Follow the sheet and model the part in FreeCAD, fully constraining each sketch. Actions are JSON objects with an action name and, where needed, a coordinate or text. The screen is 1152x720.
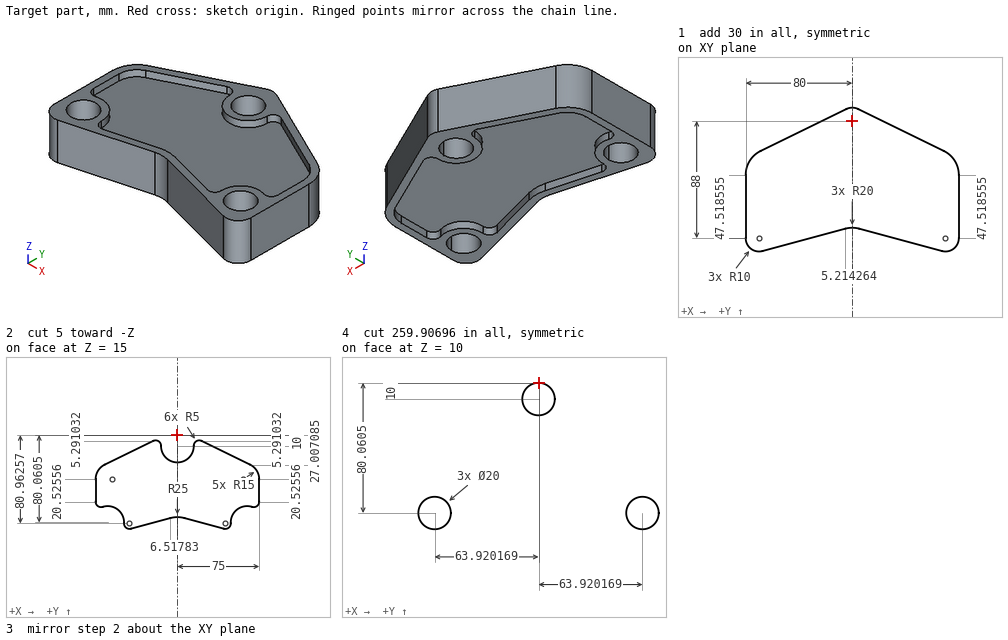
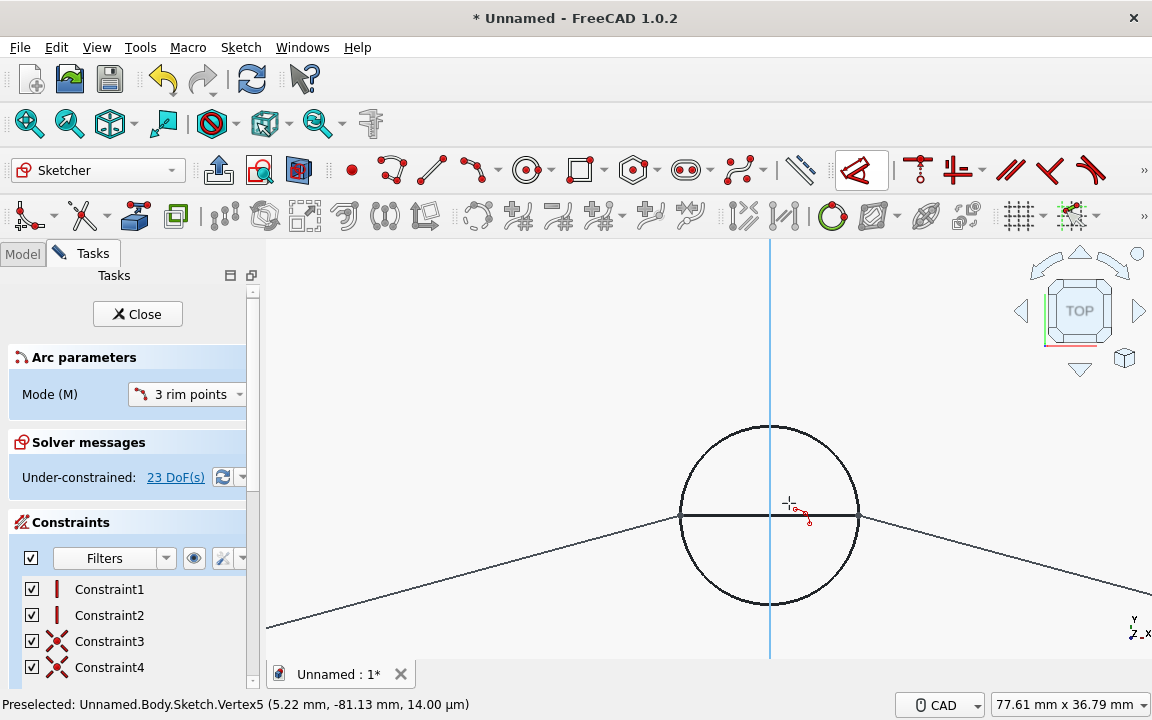
{"action": "left_click", "coordinate": [787, 498]}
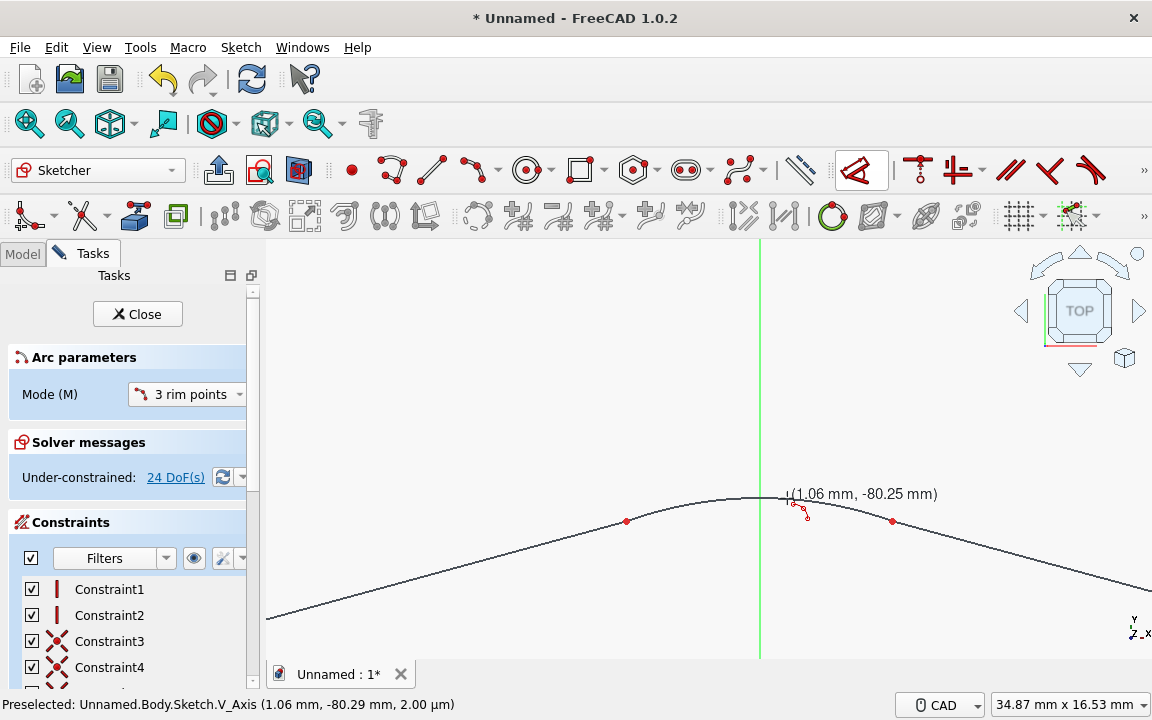
{"action": "scroll", "coordinate": [629, 536], "scroll_direction": "down", "scroll_amount": 12}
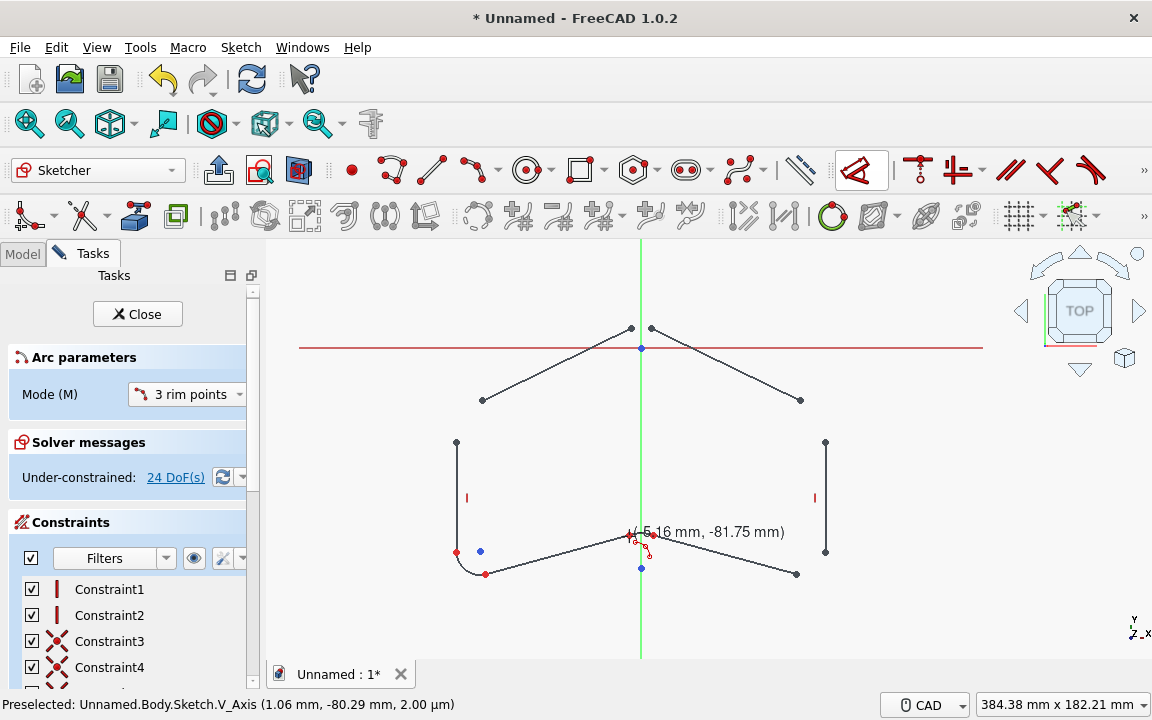
{"action": "left_click", "coordinate": [797, 574]}
{"action": "left_click", "coordinate": [826, 552]}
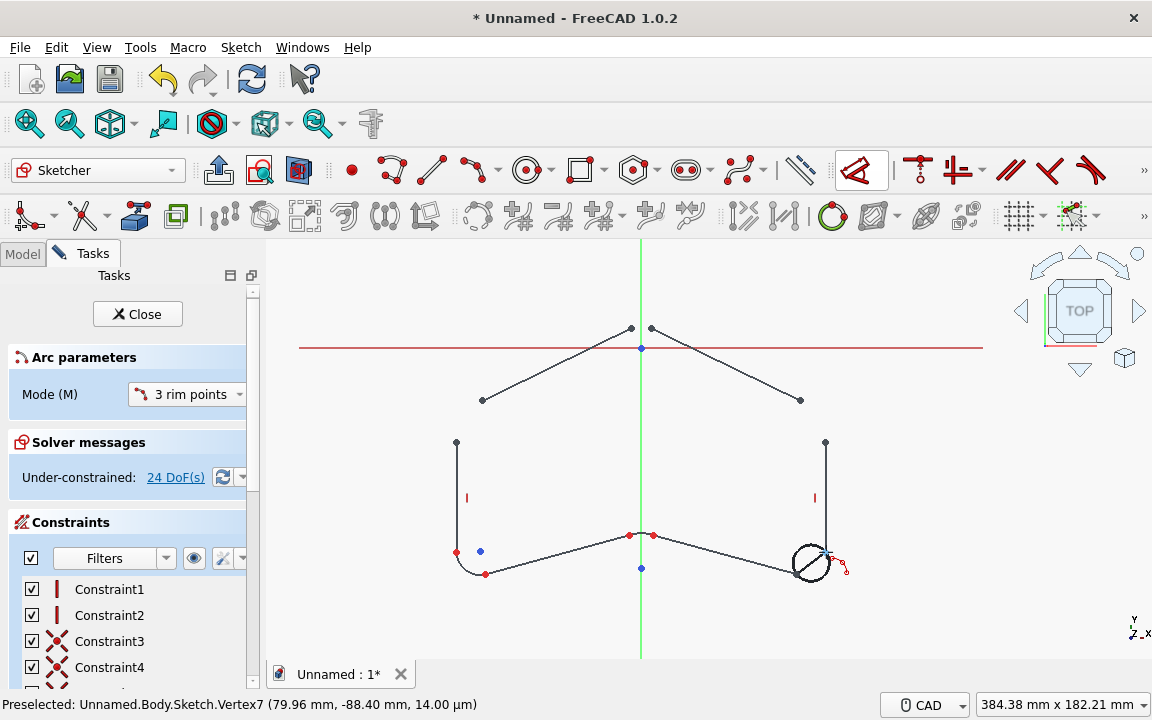
{"action": "scroll", "coordinate": [817, 569], "scroll_direction": "up", "scroll_amount": 3}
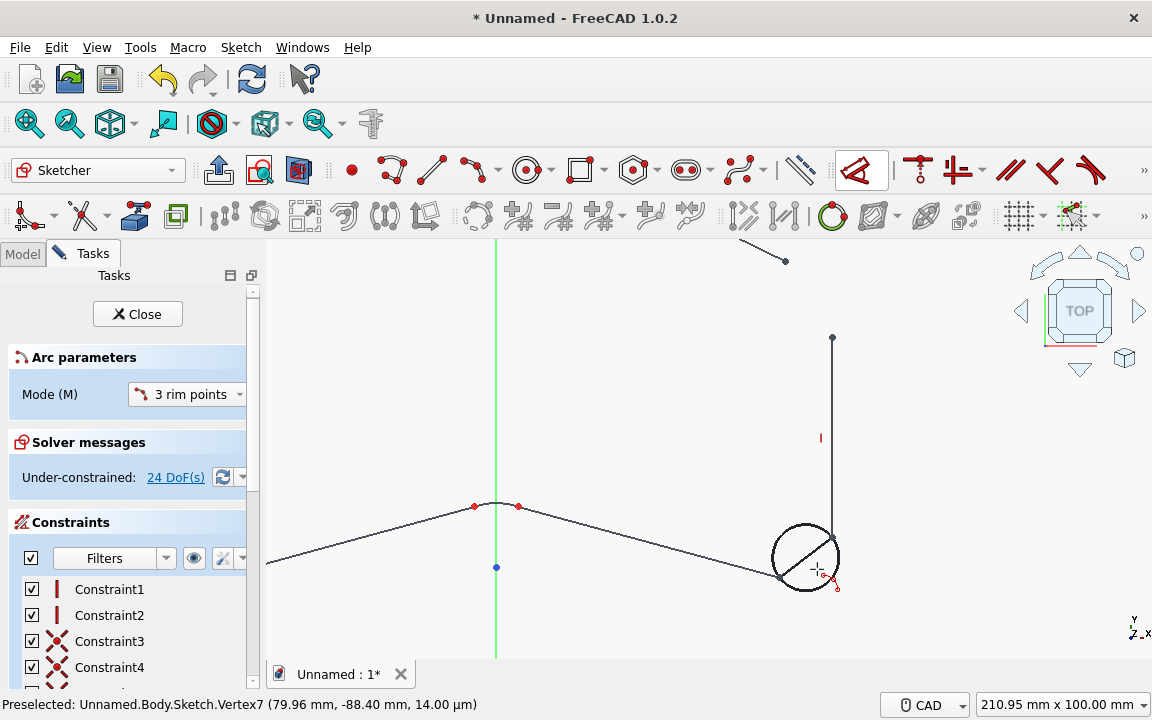
{"action": "left_click", "coordinate": [816, 569]}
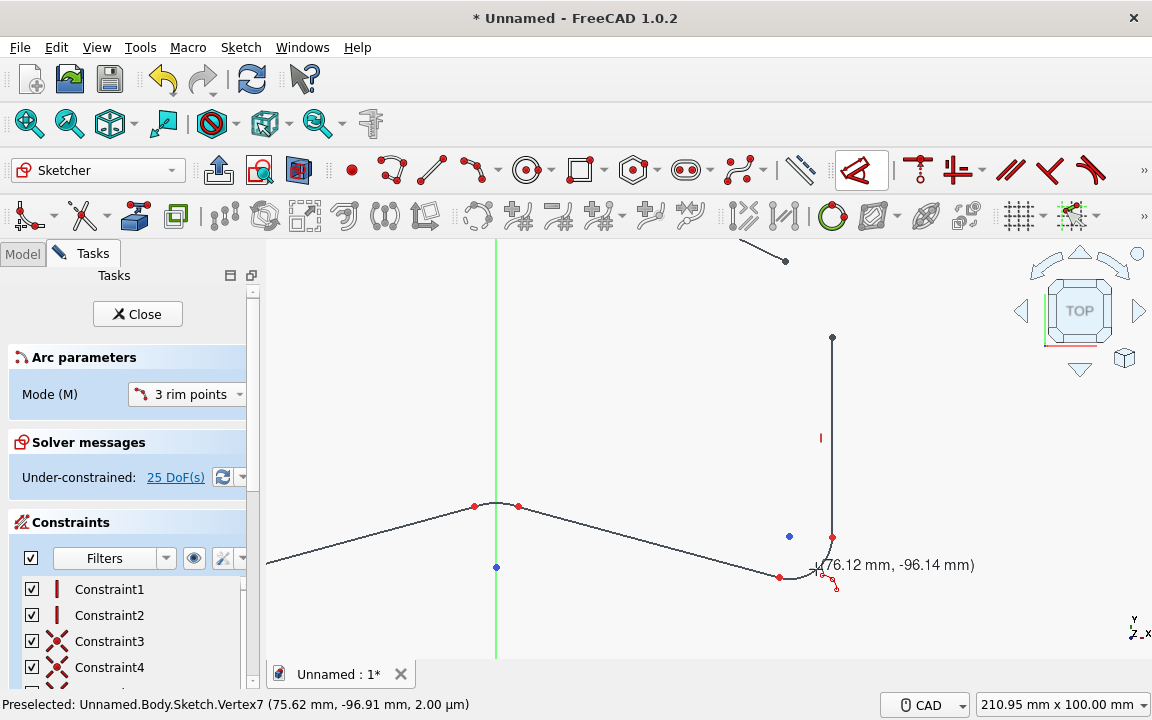
{"action": "left_click", "coordinate": [832, 337]}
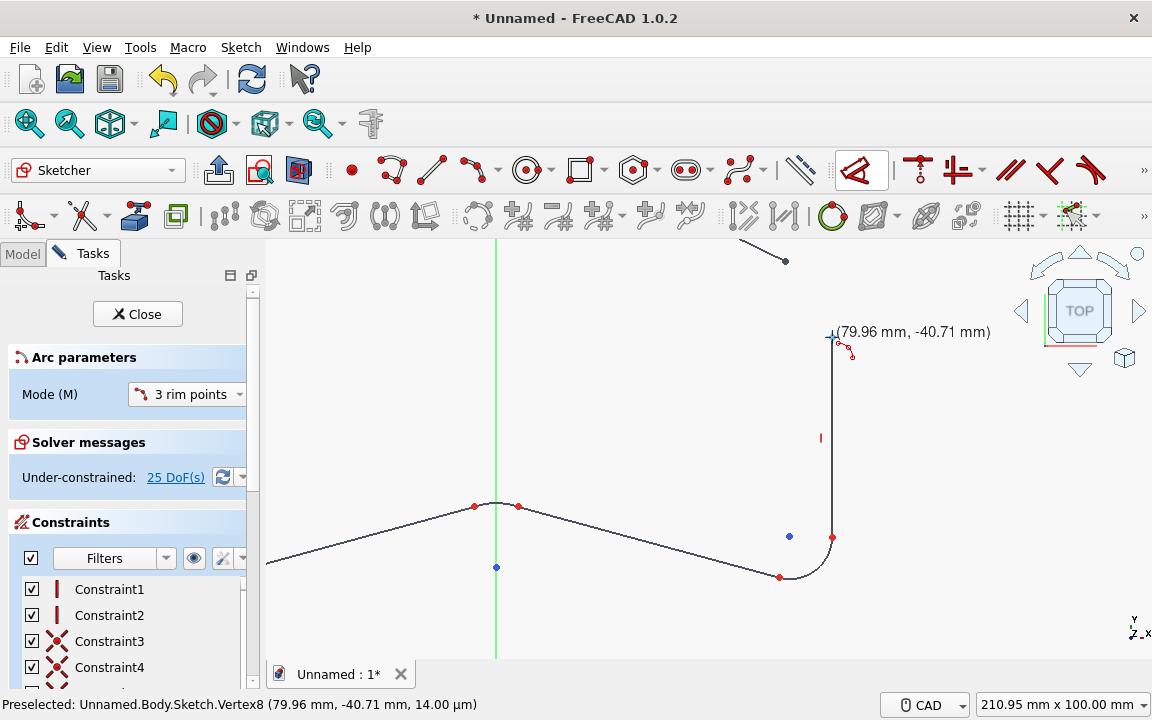
{"action": "scroll", "coordinate": [816, 569], "scroll_direction": "down", "scroll_amount": 3}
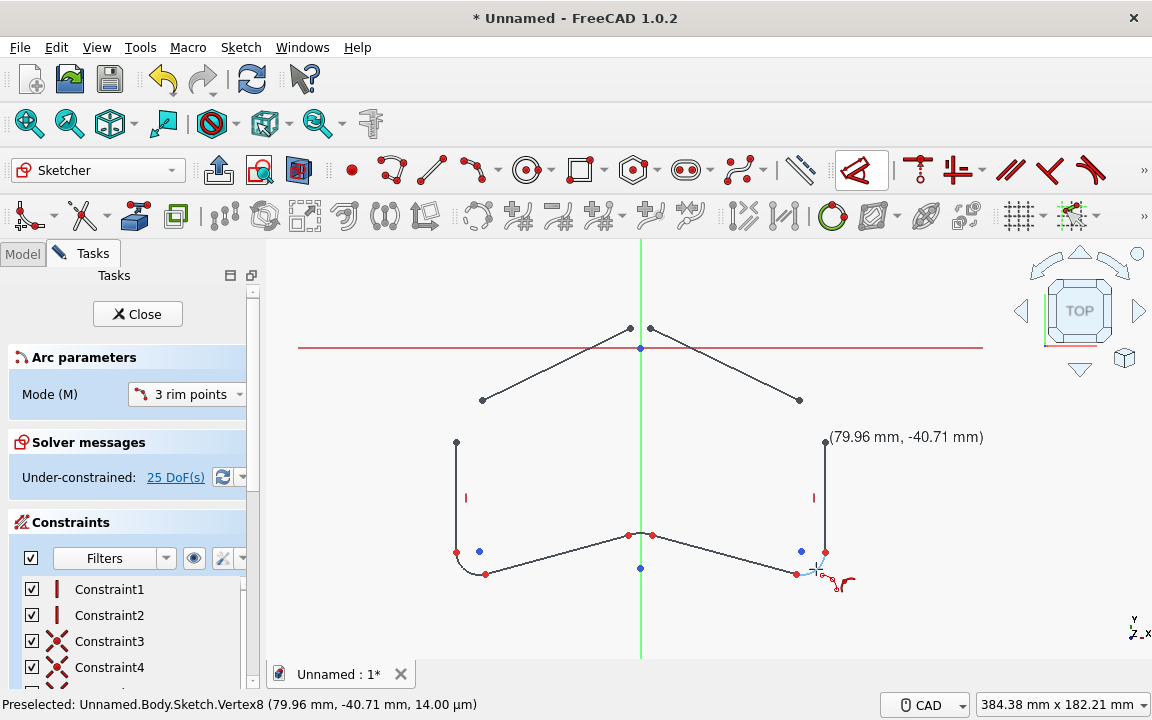
{"action": "left_click", "coordinate": [800, 401]}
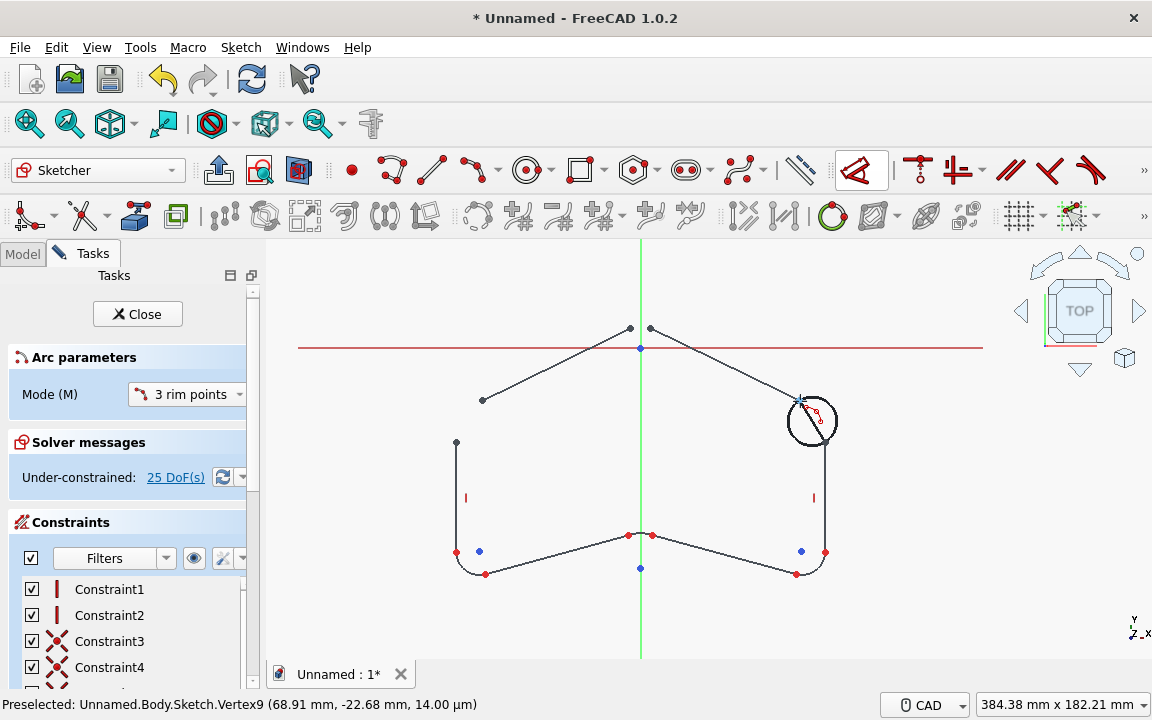
{"action": "scroll", "coordinate": [818, 417], "scroll_direction": "up", "scroll_amount": 5}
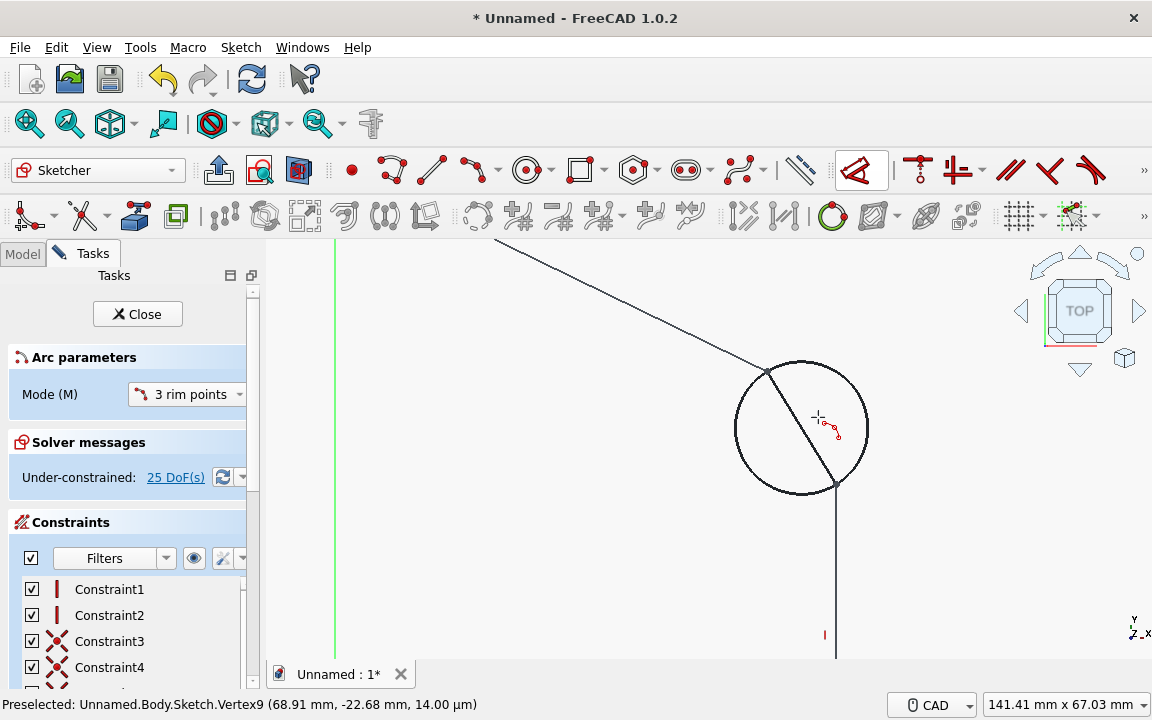
{"action": "left_click", "coordinate": [818, 417]}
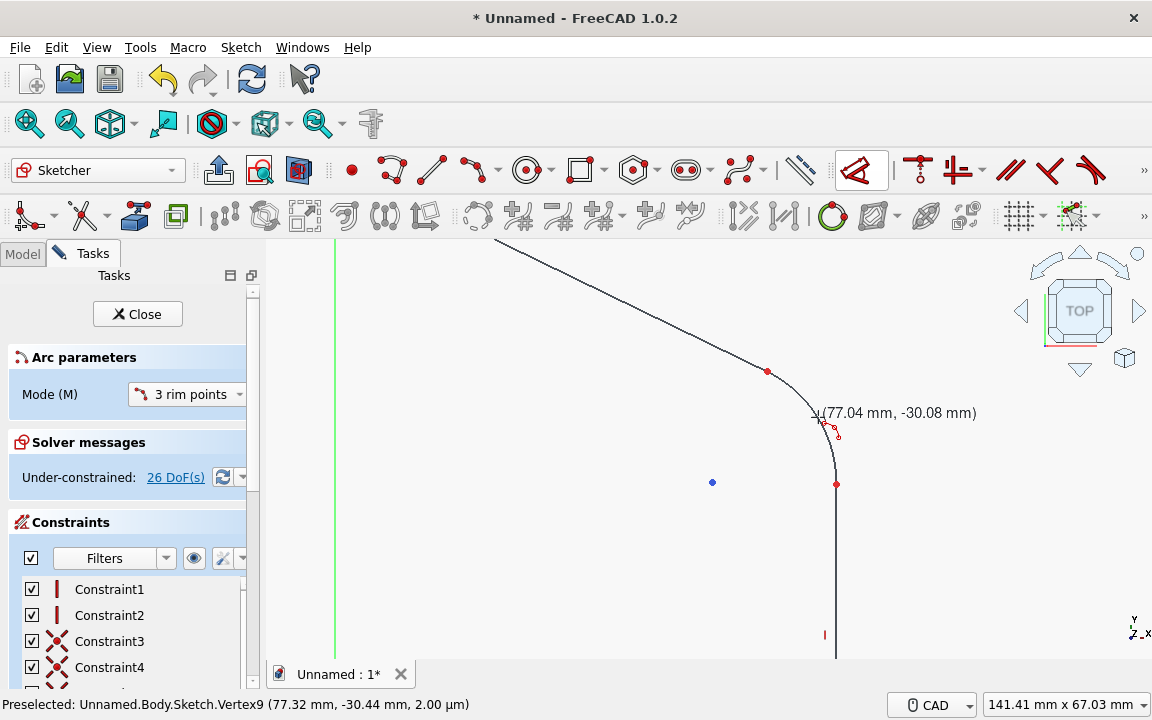
{"action": "scroll", "coordinate": [818, 417], "scroll_direction": "down", "scroll_amount": 5}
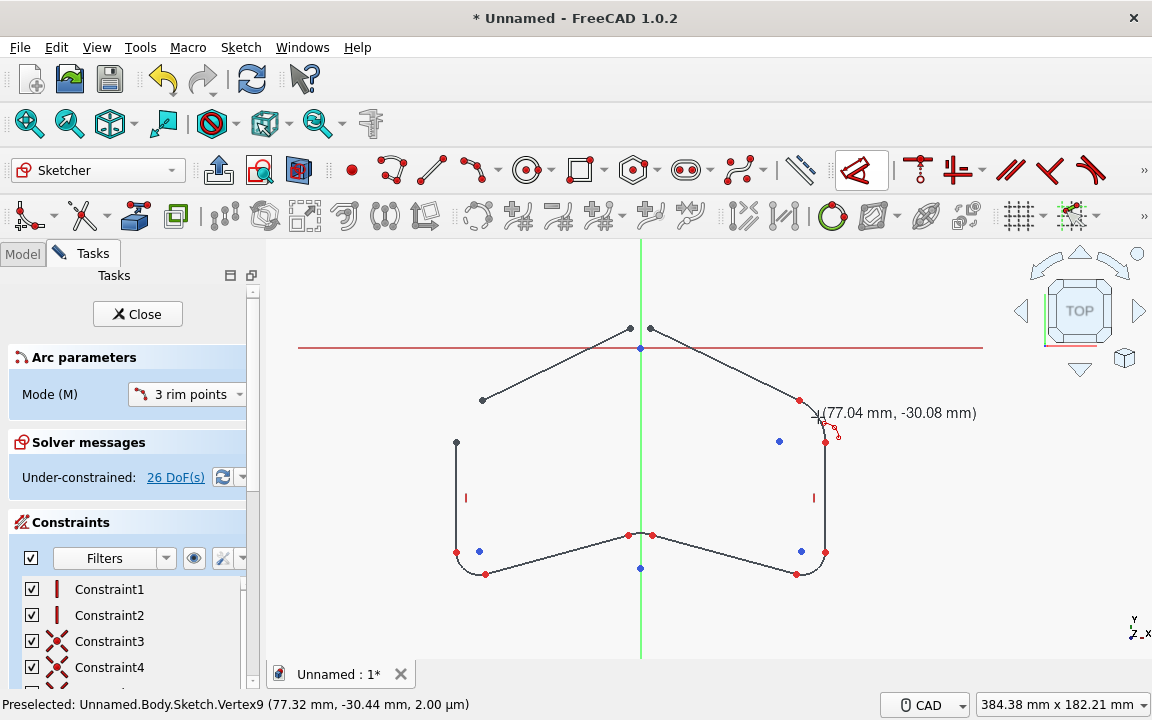
{"action": "scroll", "coordinate": [651, 328], "scroll_direction": "up", "scroll_amount": 3}